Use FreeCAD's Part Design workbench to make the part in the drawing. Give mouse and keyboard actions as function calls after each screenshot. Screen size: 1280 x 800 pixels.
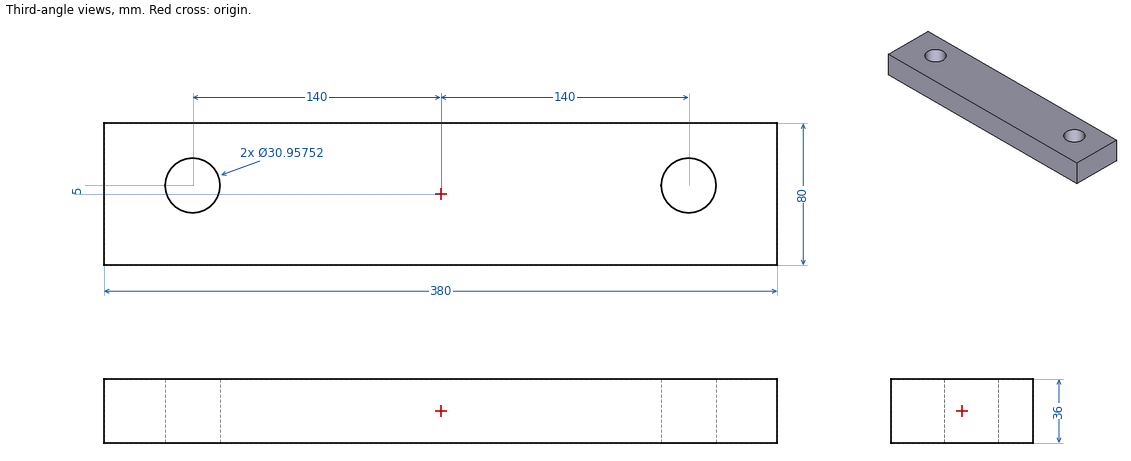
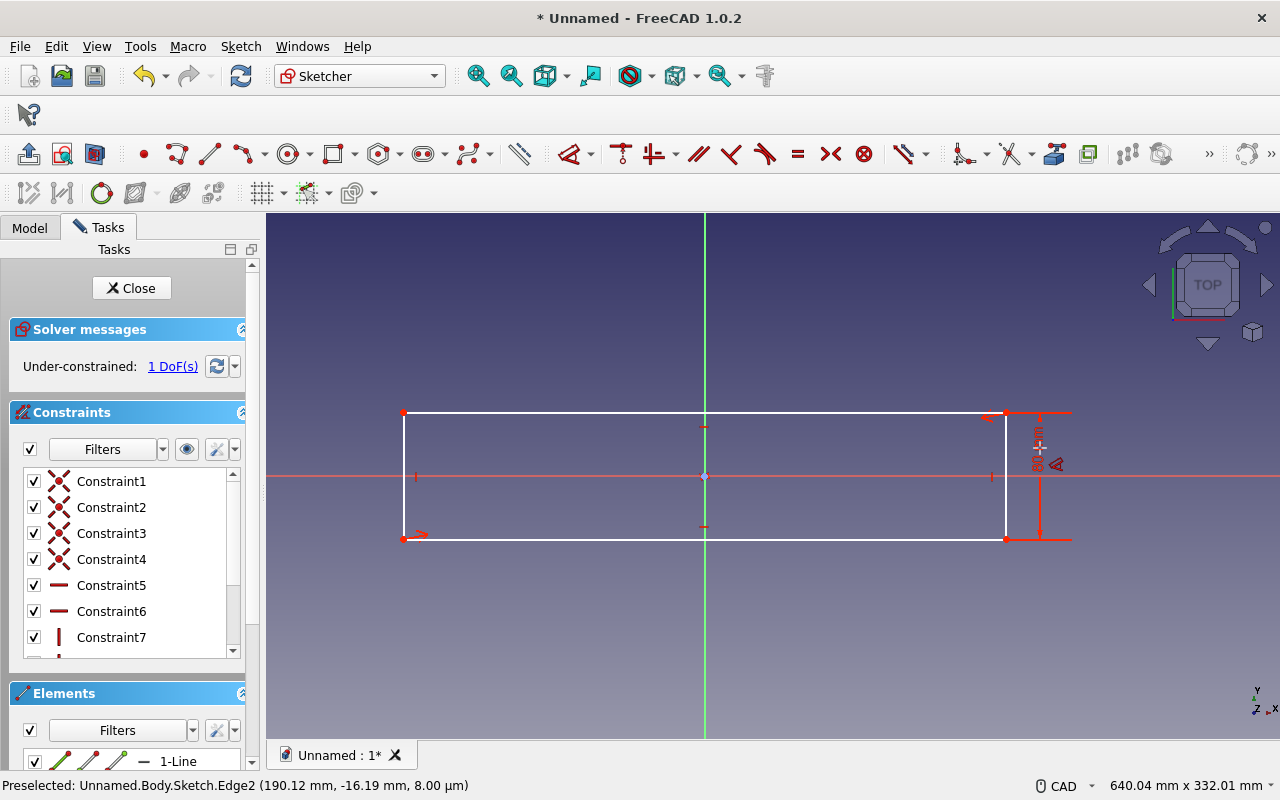
click(584, 540)
click(566, 574)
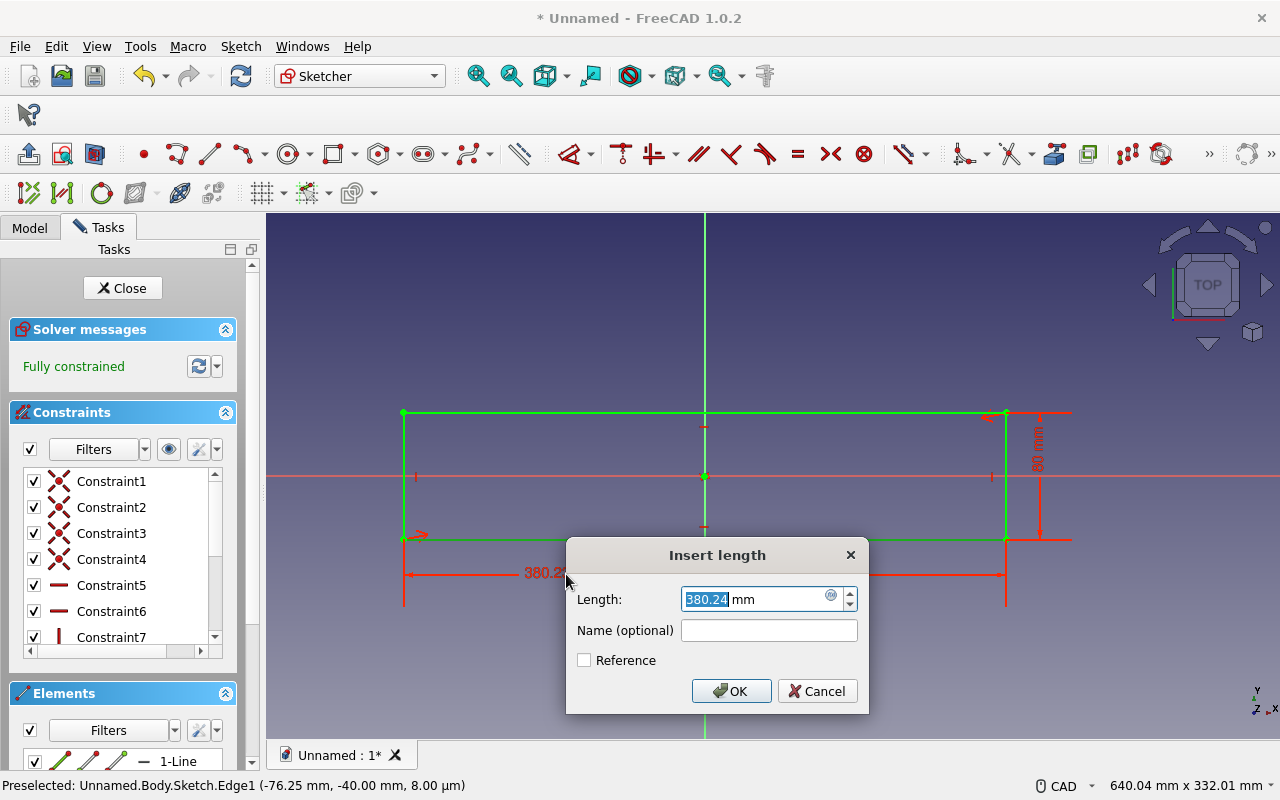
text(380)
key(Return)
key(Escape)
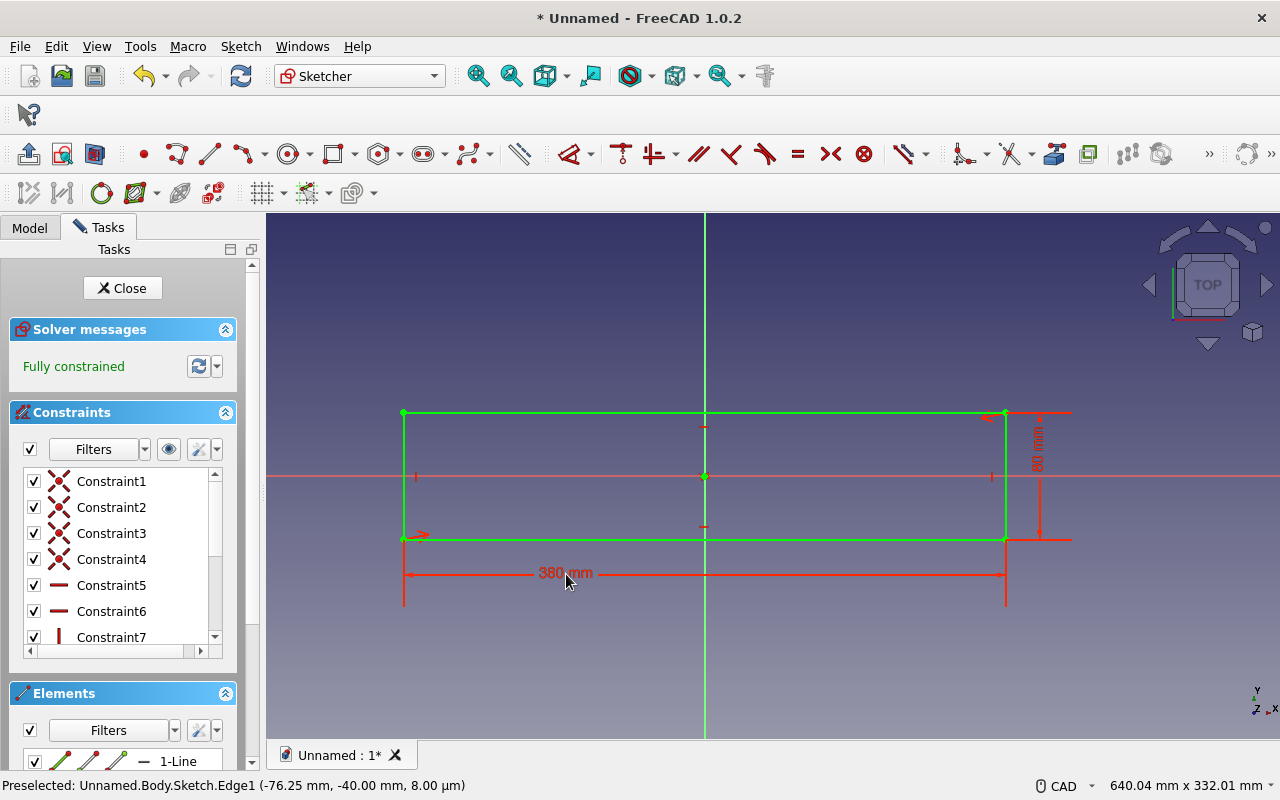
click(123, 288)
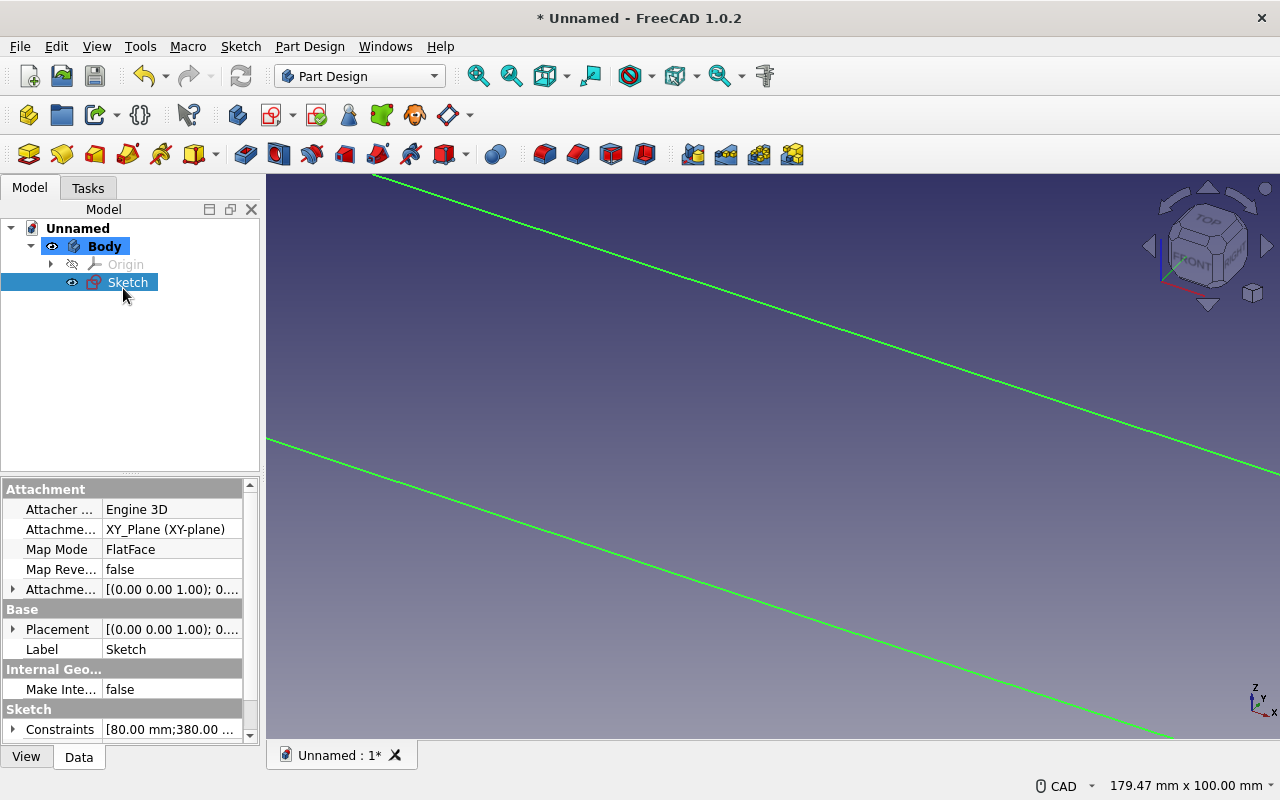
click(29, 154)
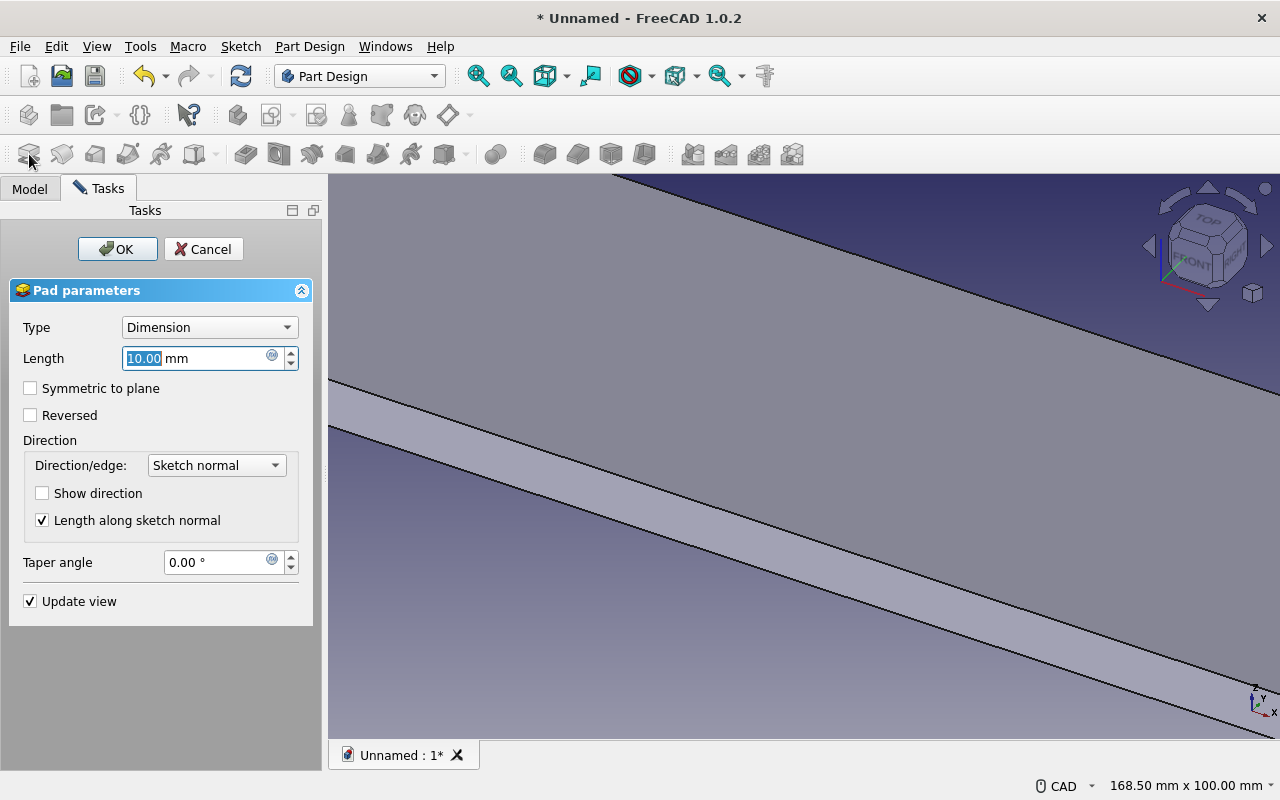
text(36)
key(Tab)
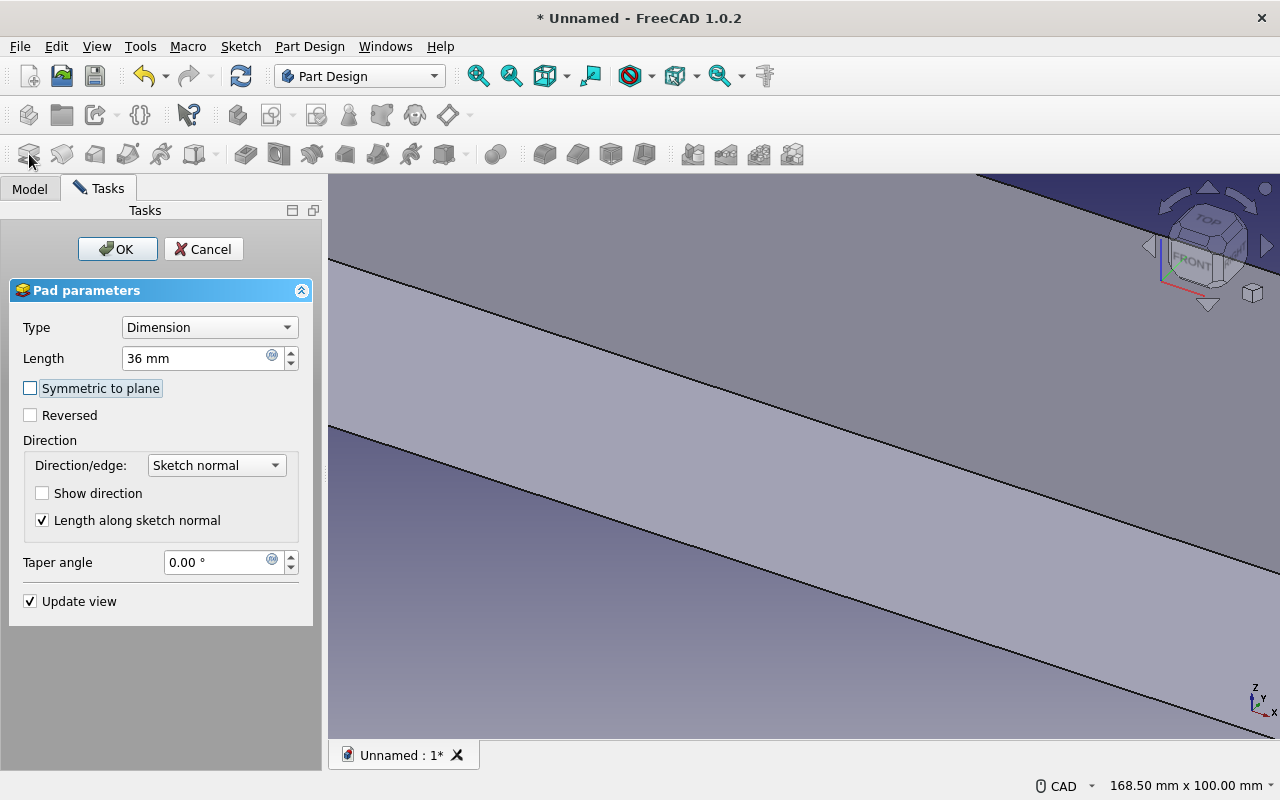
click(31, 388)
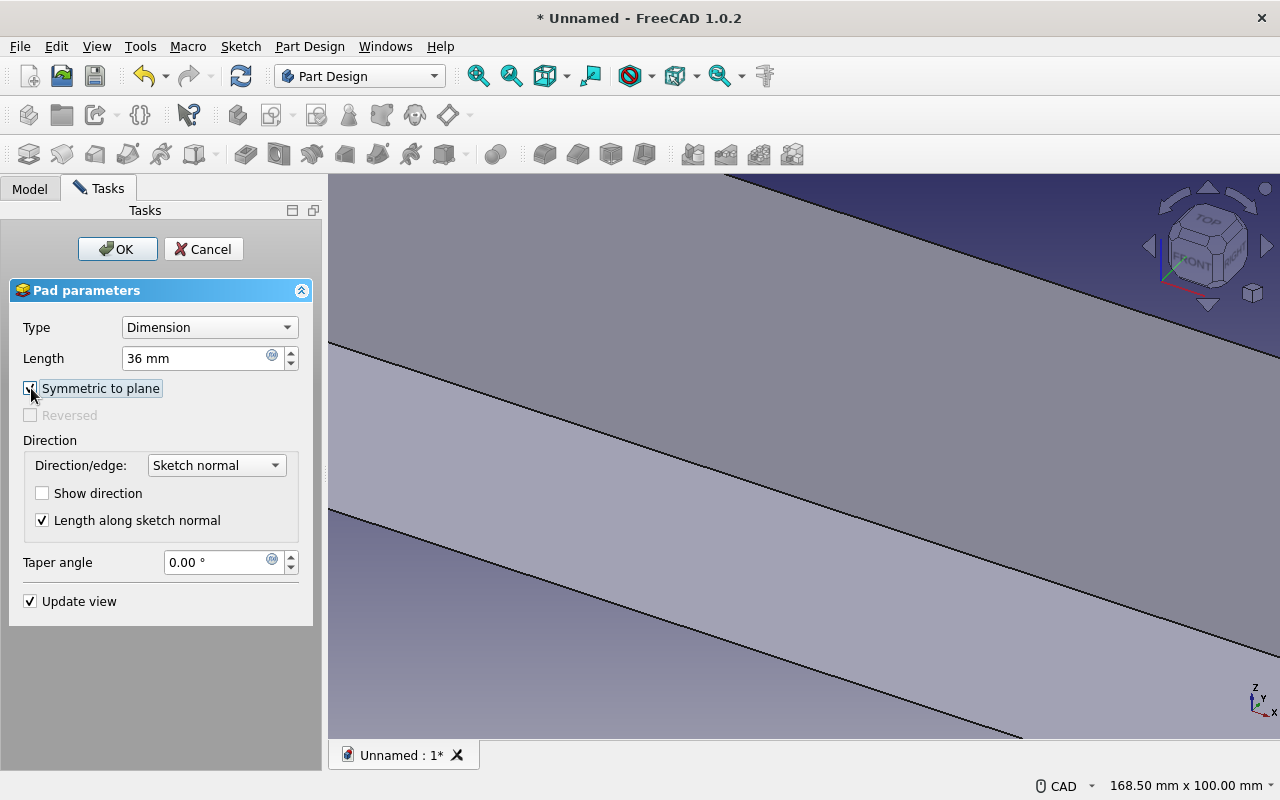
click(118, 249)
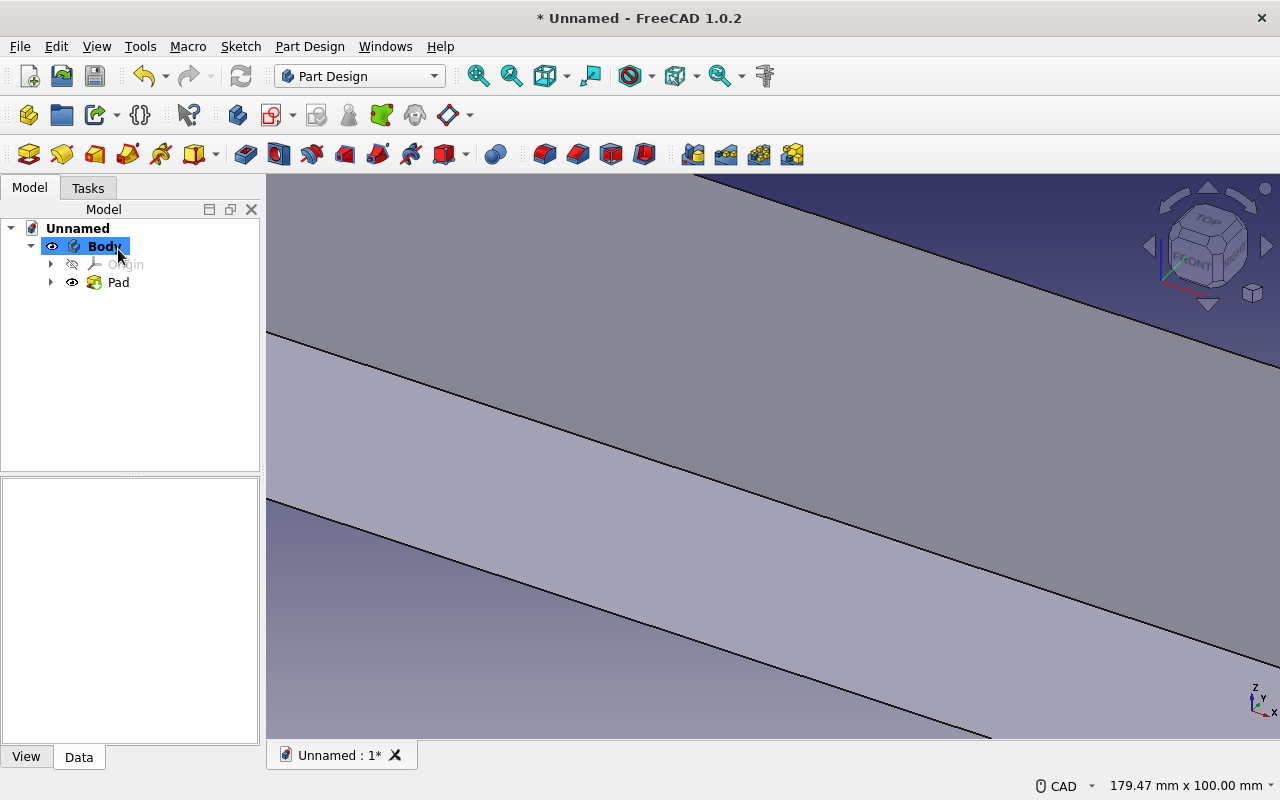
click(479, 76)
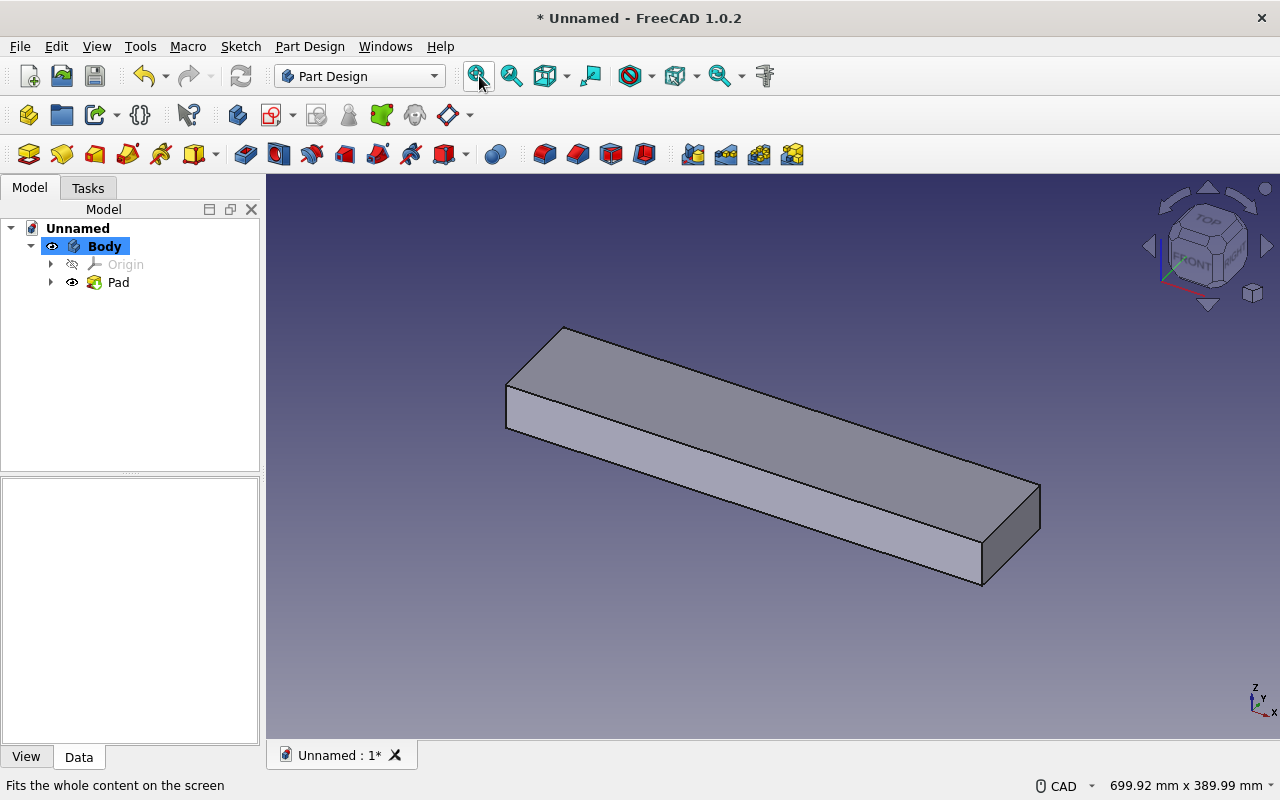
click(909, 479)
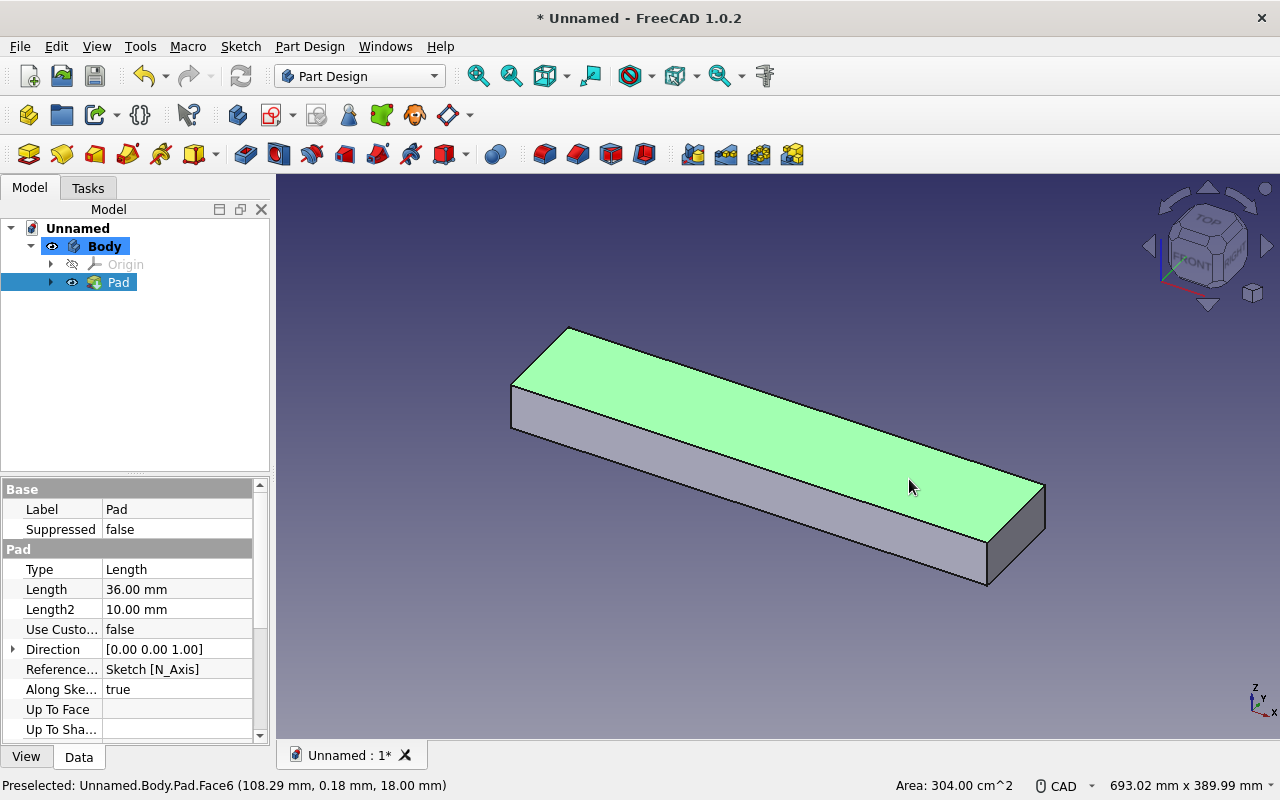
click(270, 116)